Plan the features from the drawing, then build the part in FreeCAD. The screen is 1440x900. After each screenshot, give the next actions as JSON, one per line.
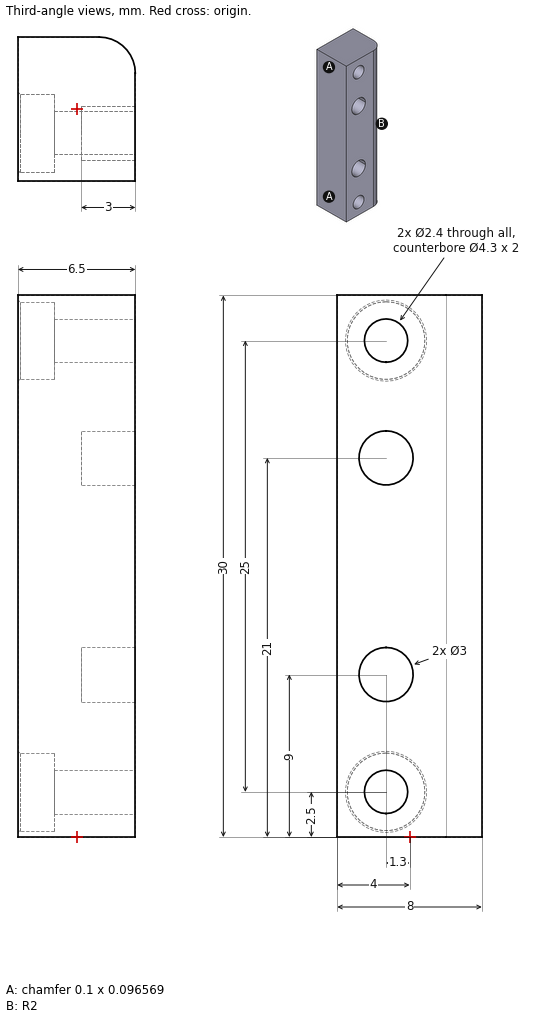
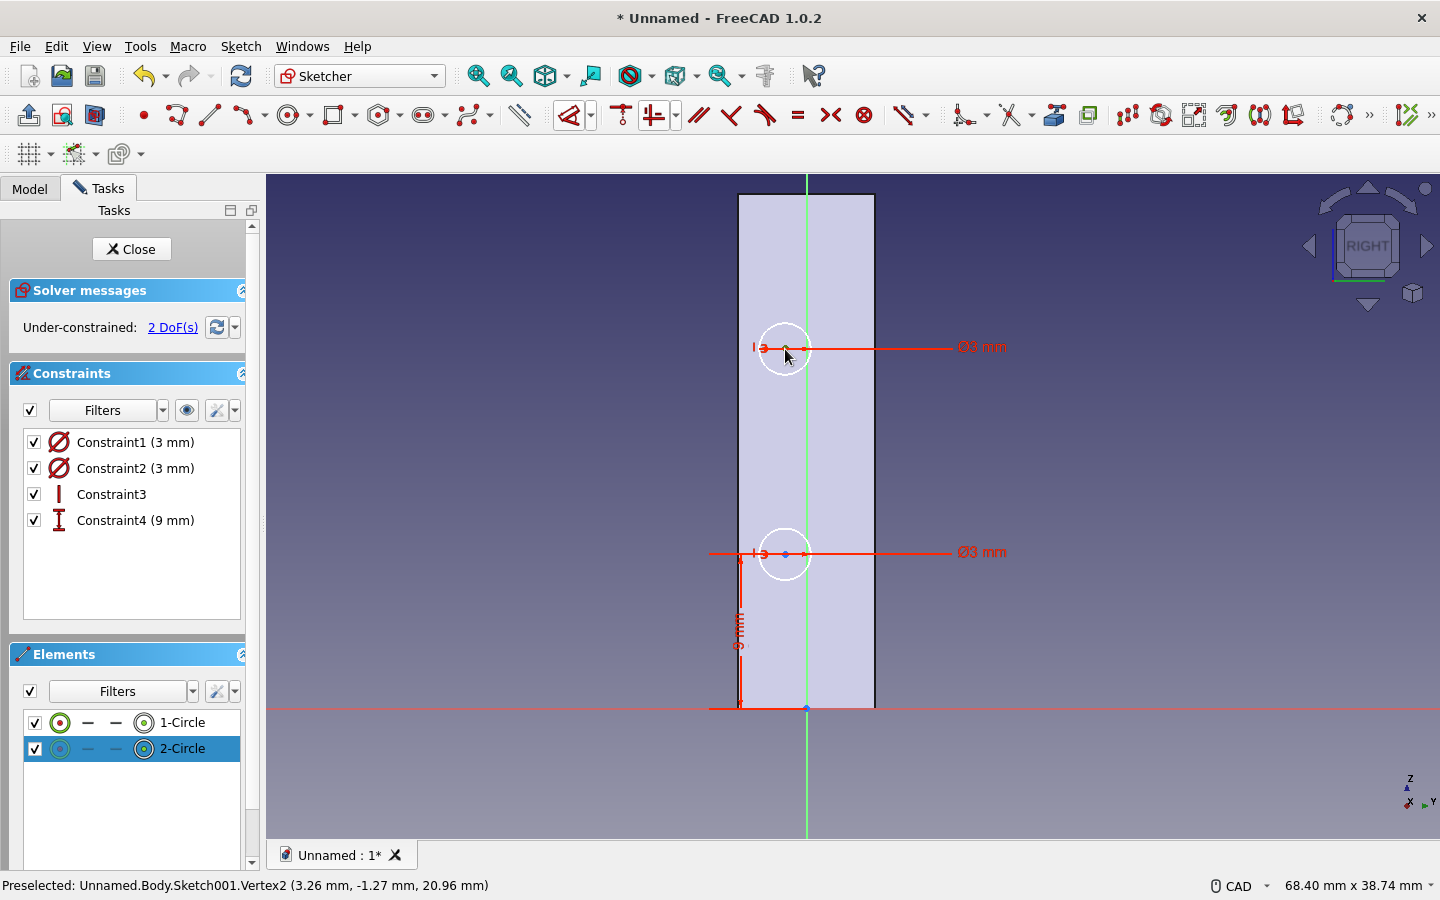
{"action": "key", "text": "i"}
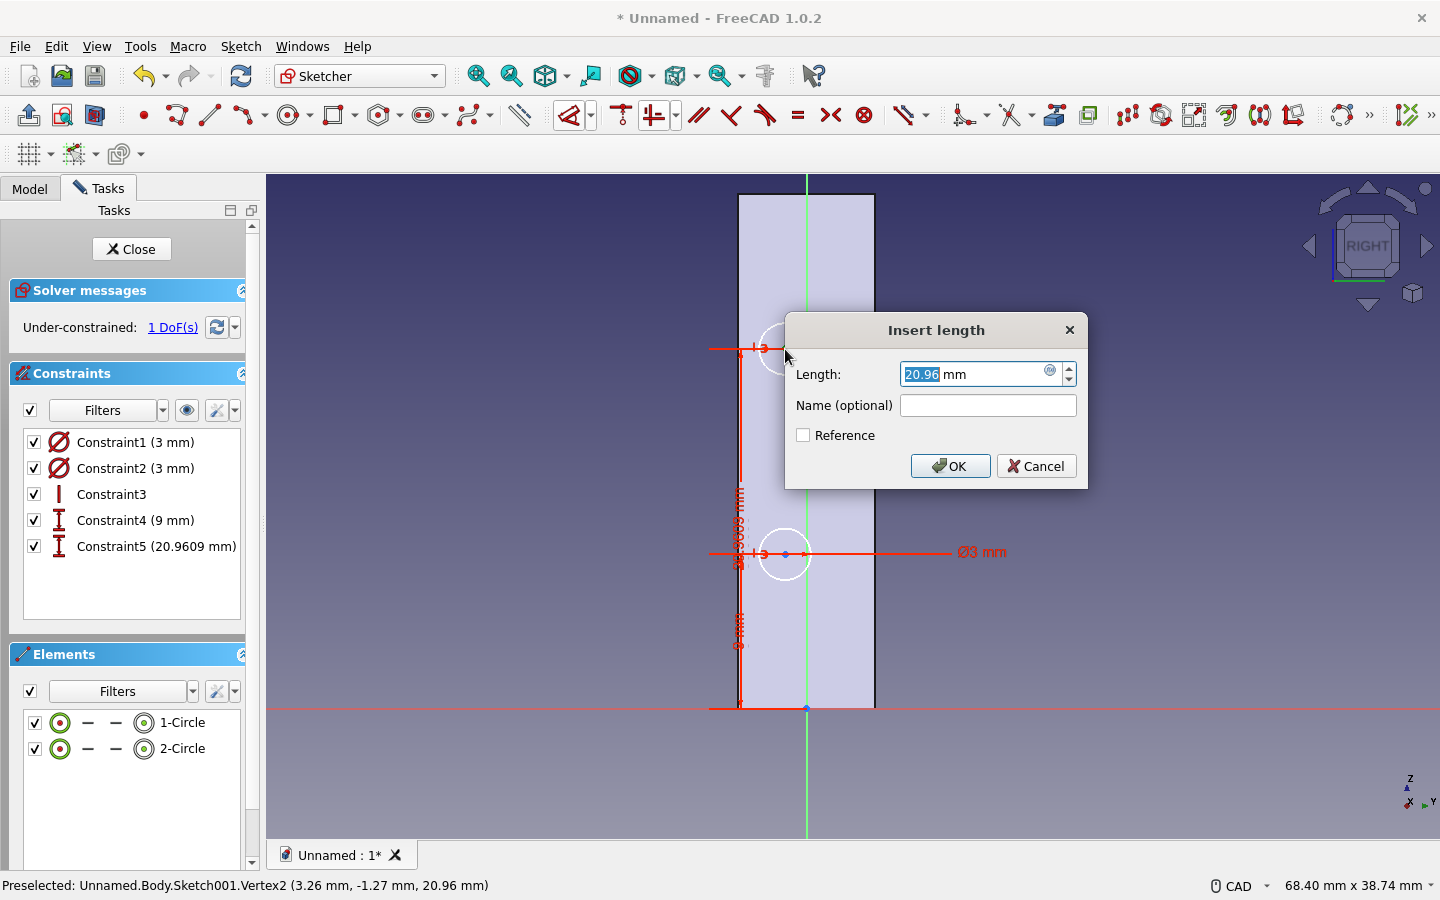
{"action": "type", "text": "21"}
{"action": "key", "text": "Return"}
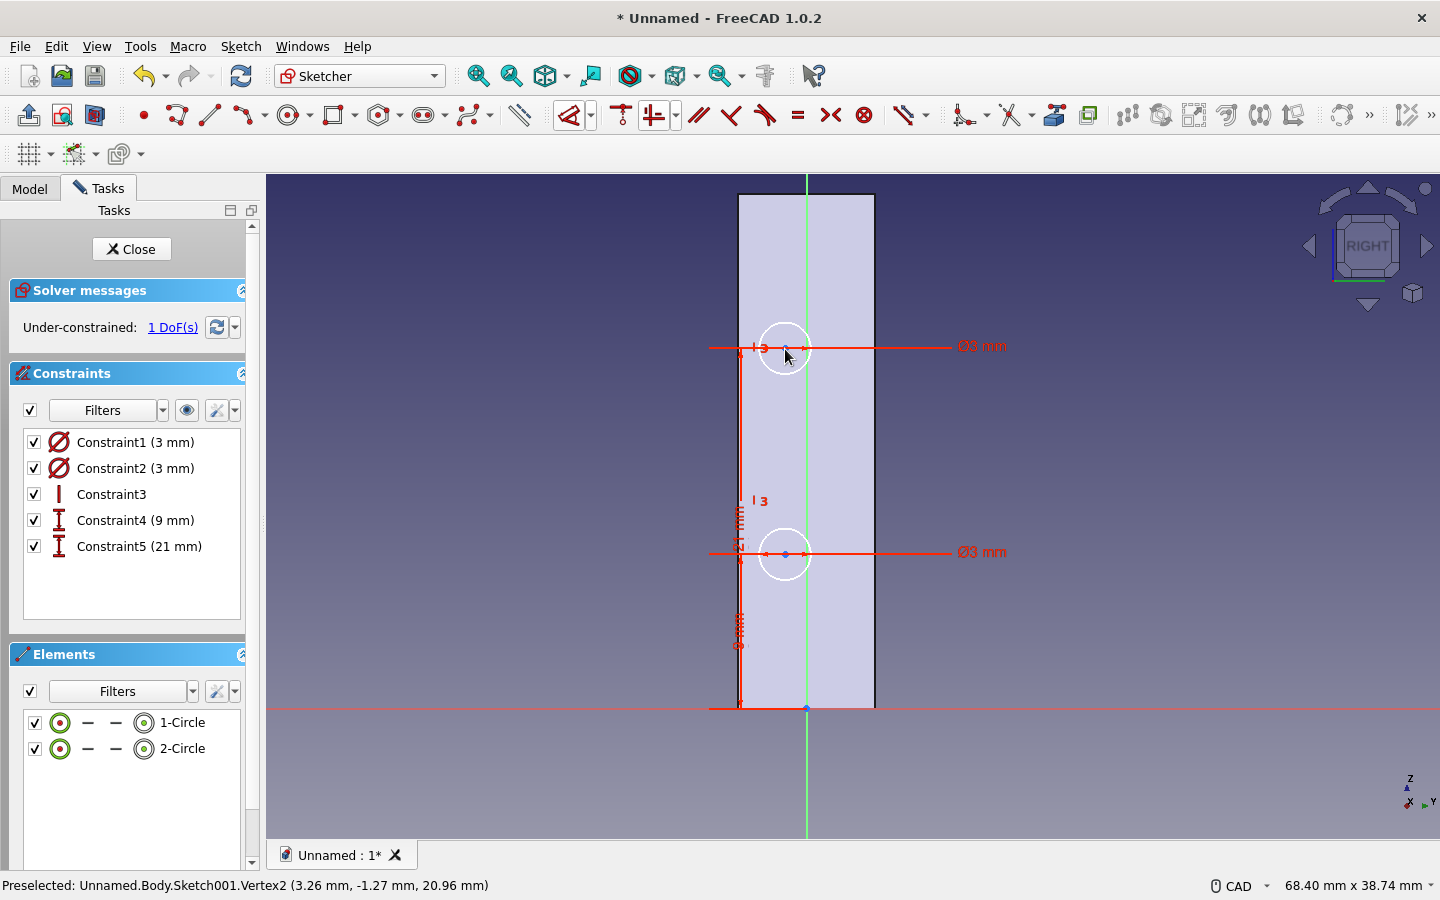
{"action": "scroll", "coordinate": [785, 554], "scroll_direction": "up", "scroll_amount": 3}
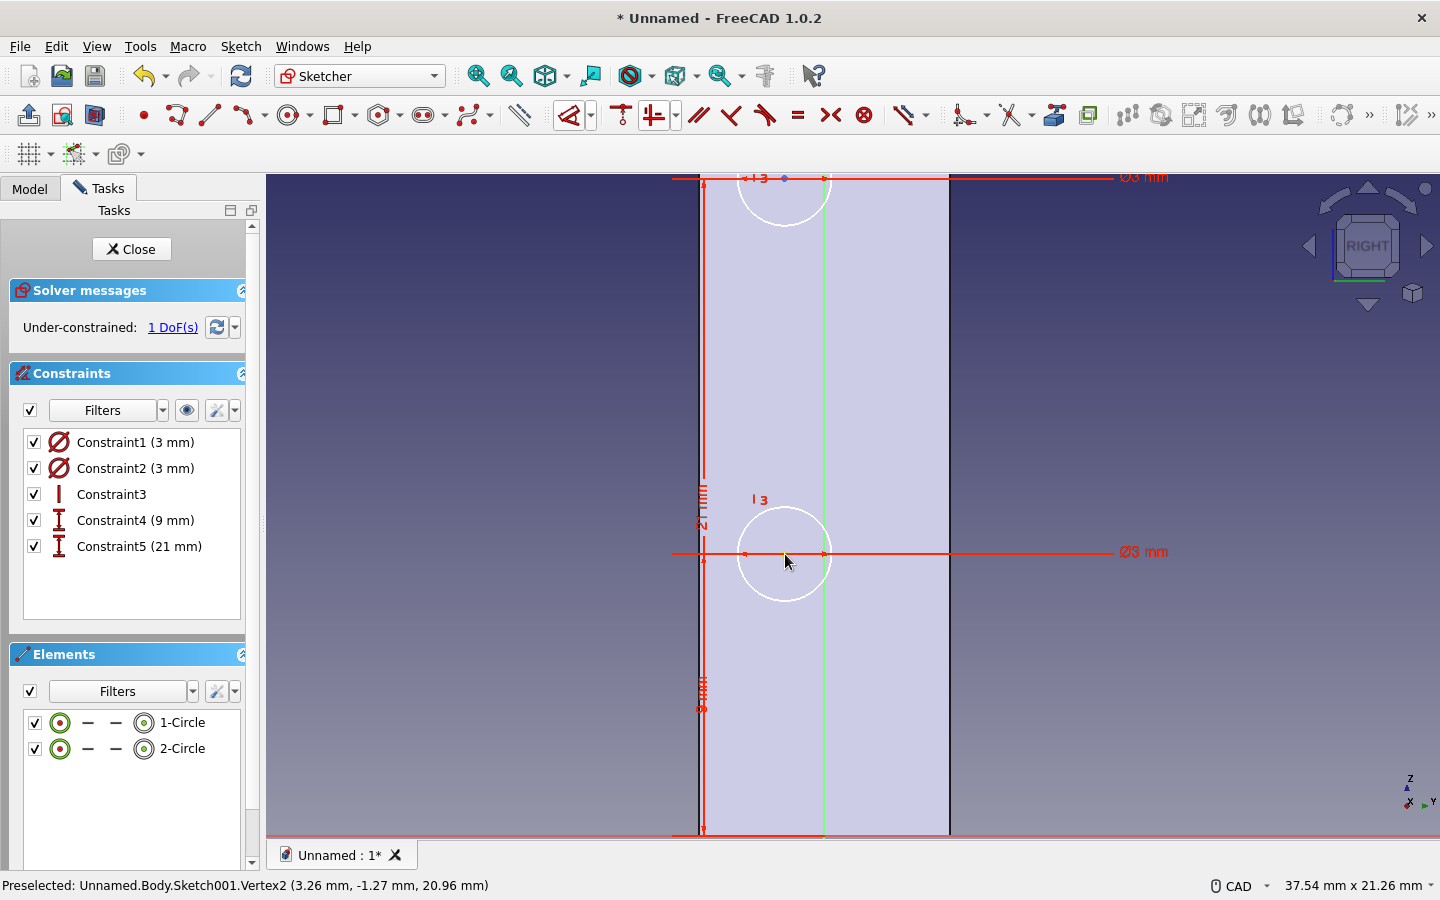
{"action": "left_click", "coordinate": [785, 554]}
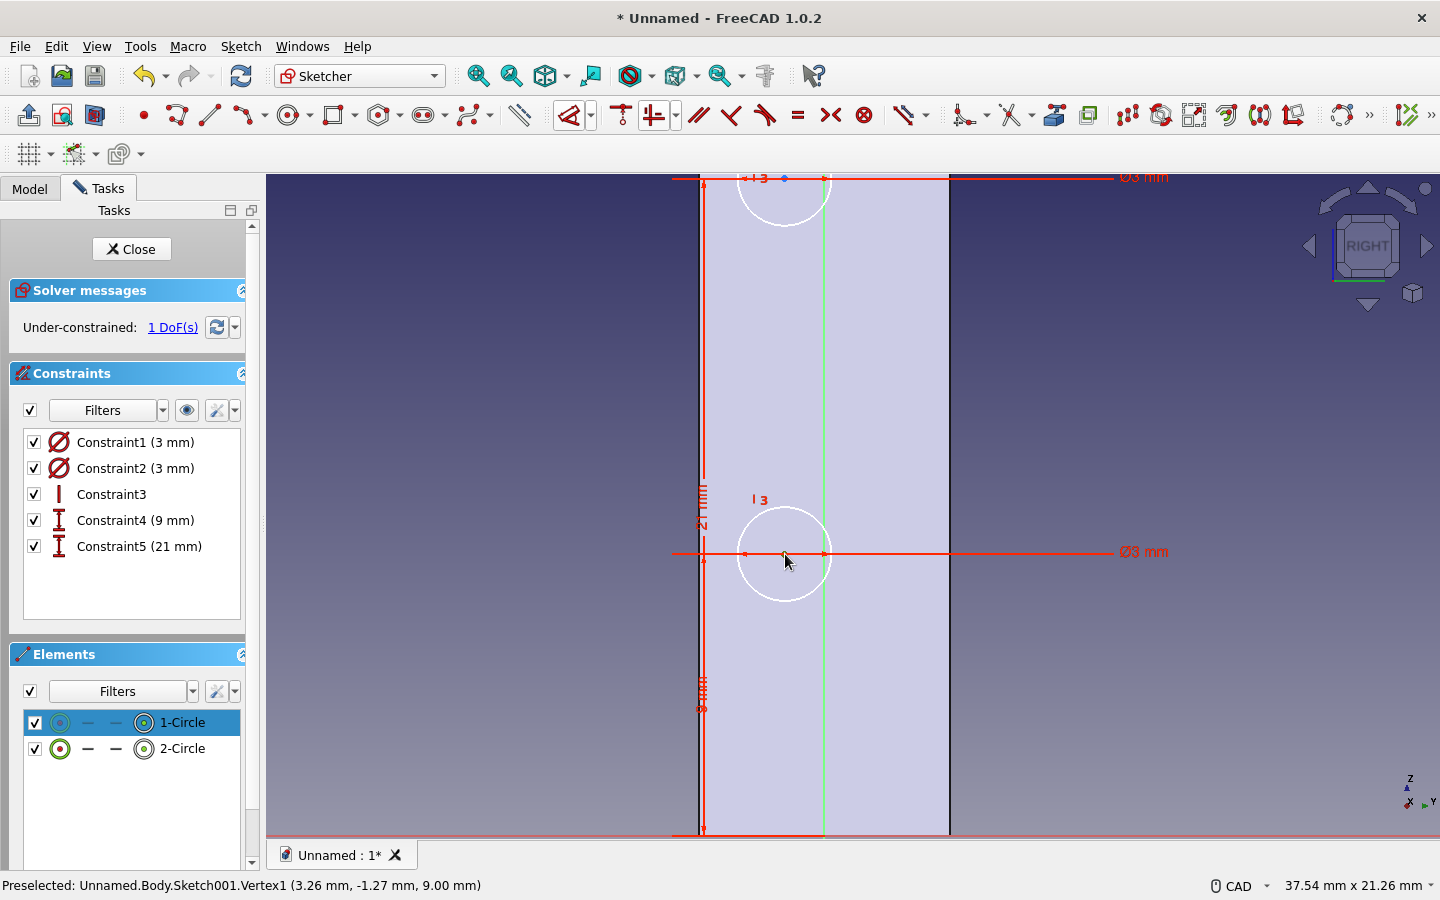
{"action": "key", "text": "l"}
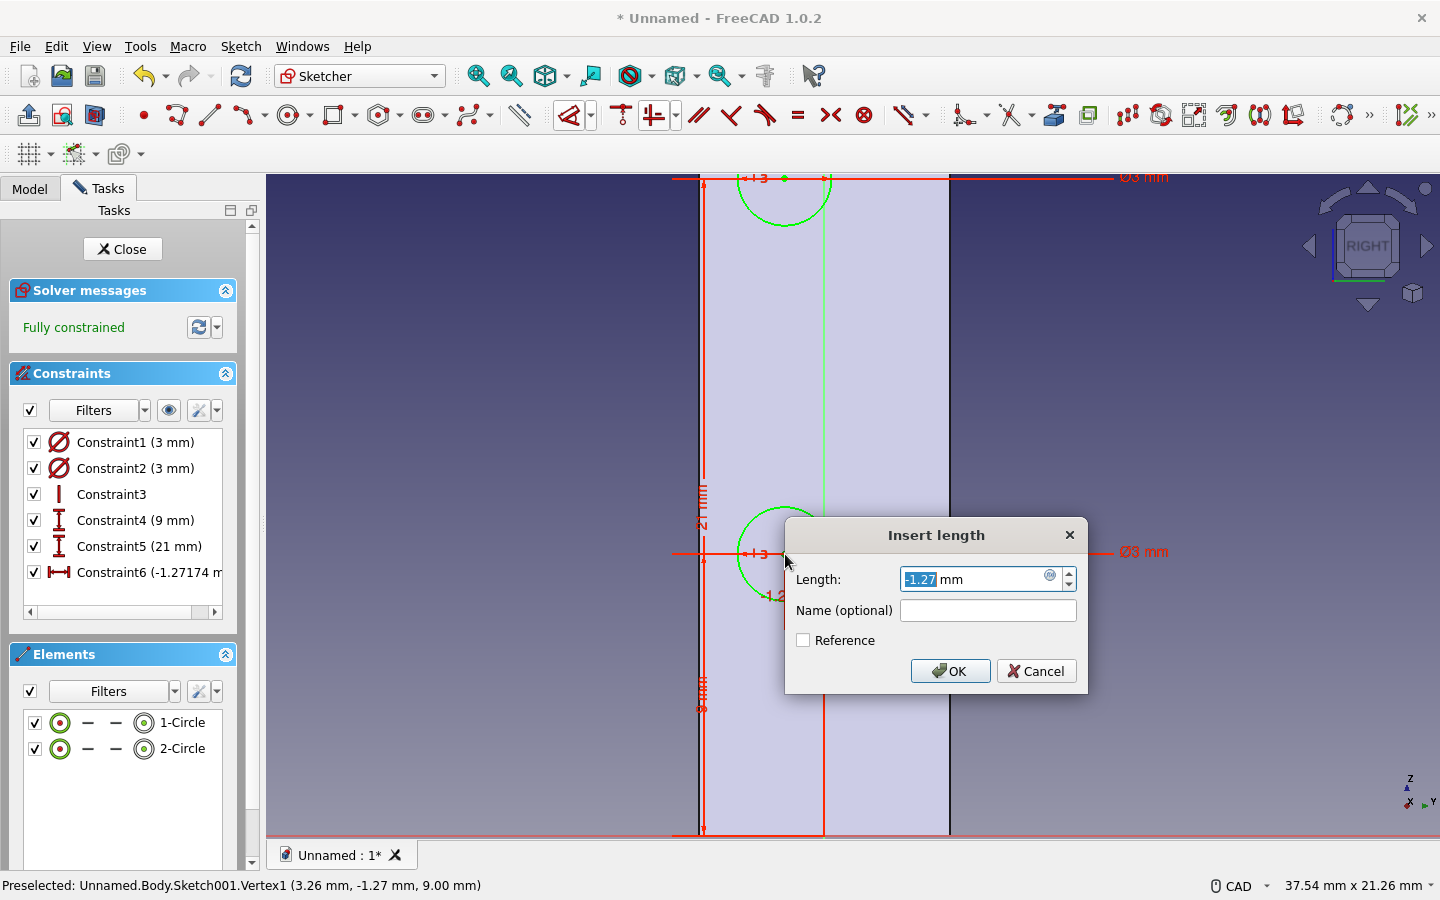
{"action": "type", "text": "-1.3"}
{"action": "key", "text": "Return"}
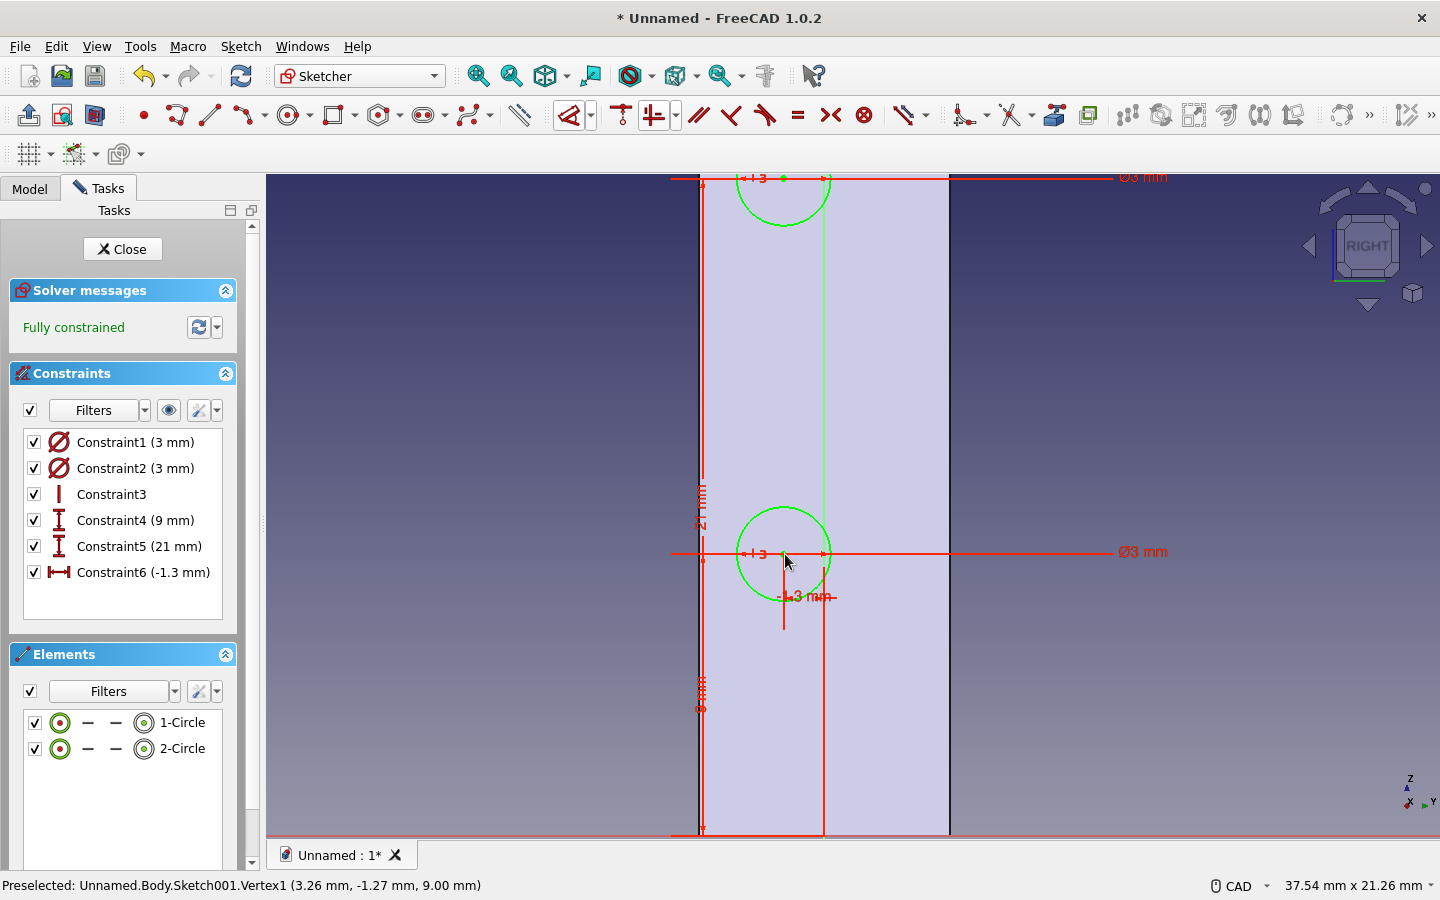
{"action": "left_click", "coordinate": [123, 249]}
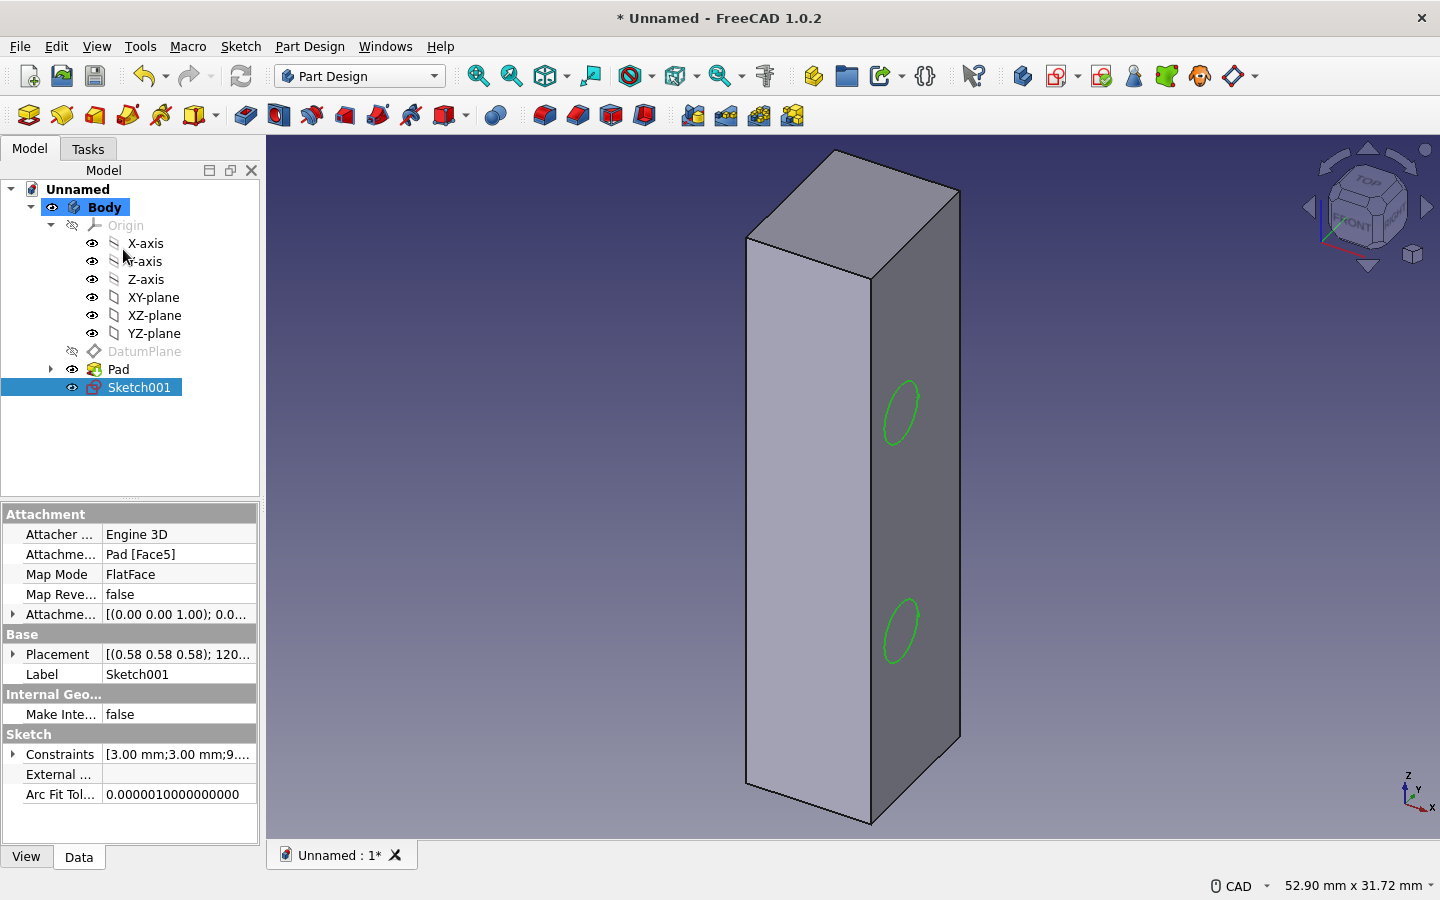
{"action": "left_click", "coordinate": [246, 116]}